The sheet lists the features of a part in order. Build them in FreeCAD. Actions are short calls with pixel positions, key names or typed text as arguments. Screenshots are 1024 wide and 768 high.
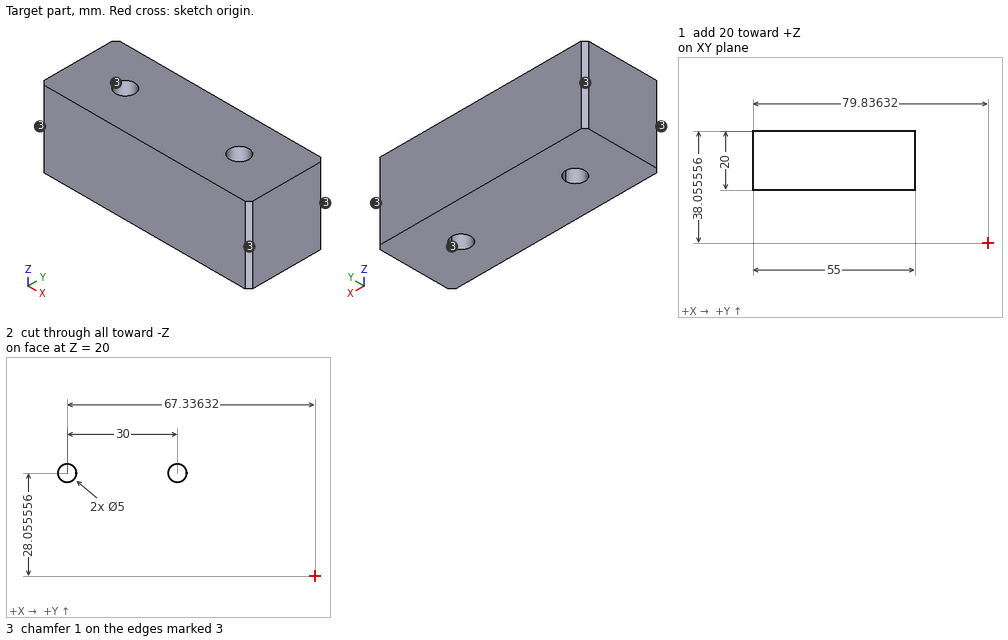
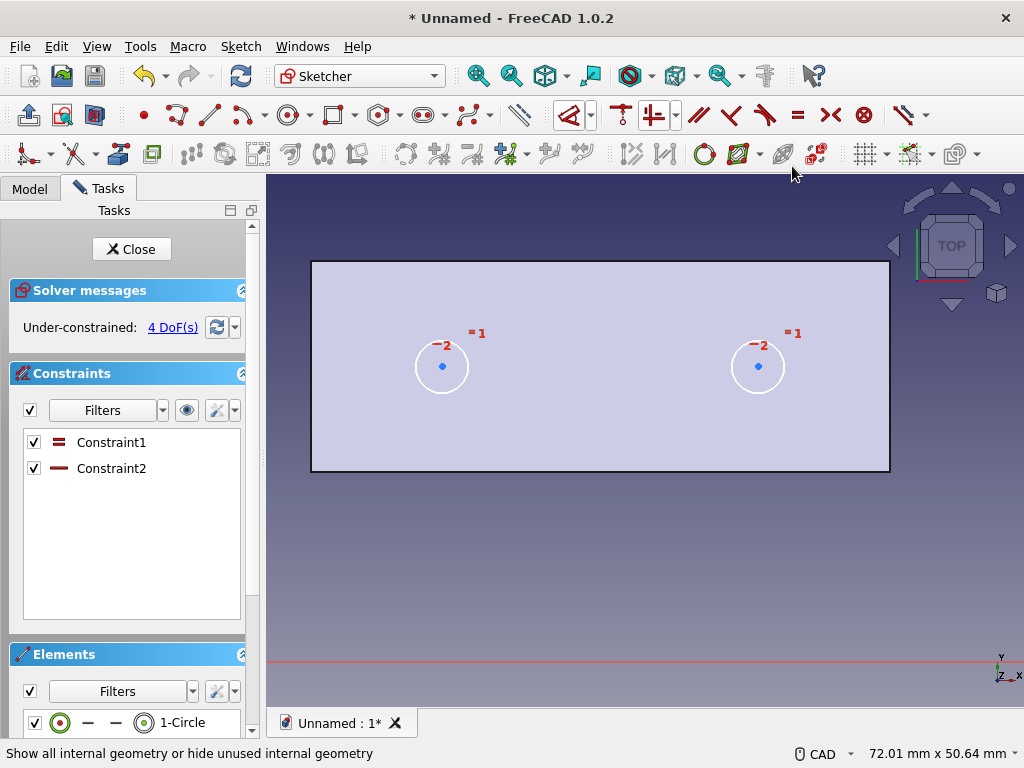
click(460, 348)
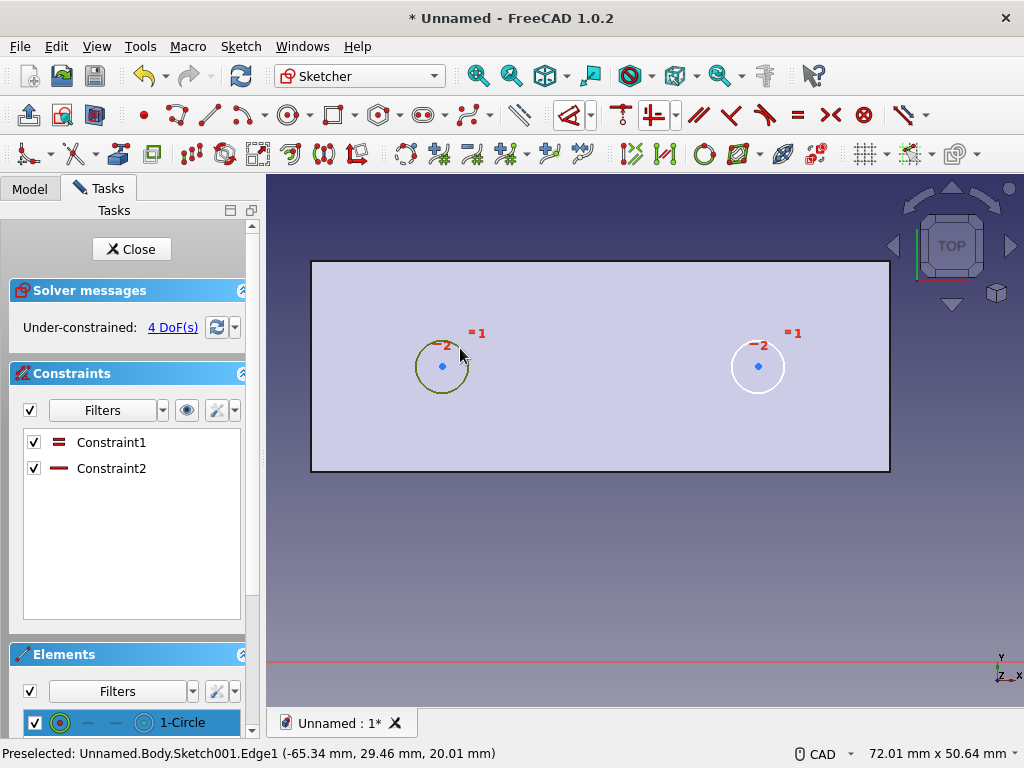
key(k)
key(o)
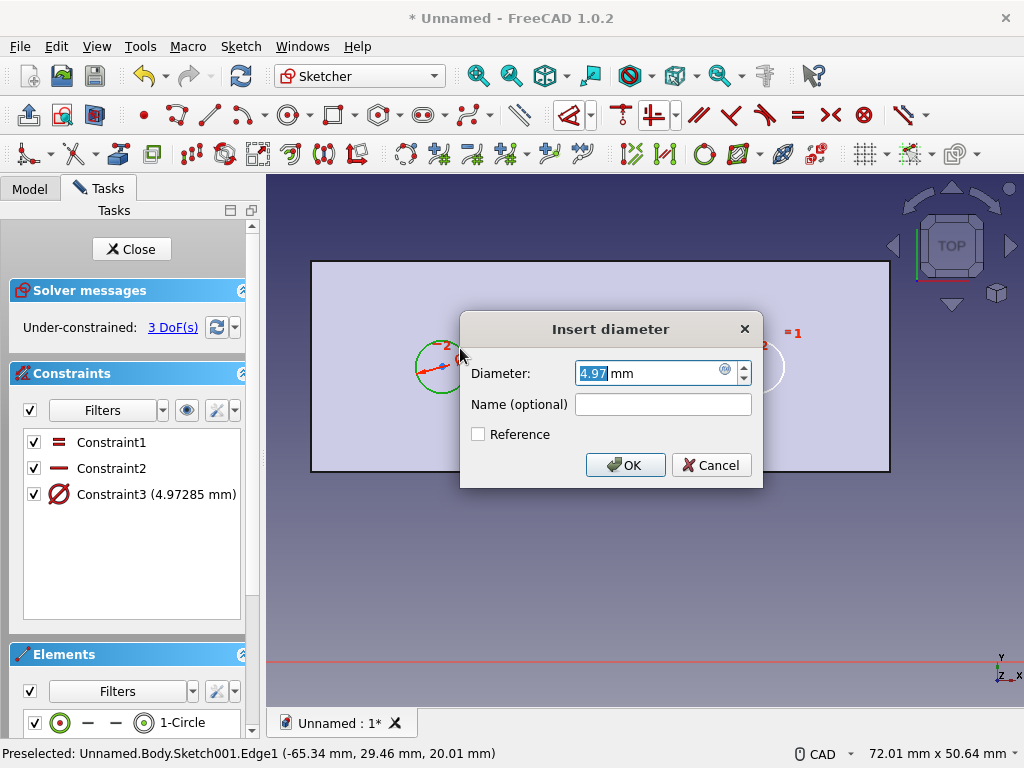
text(5)
key(Return)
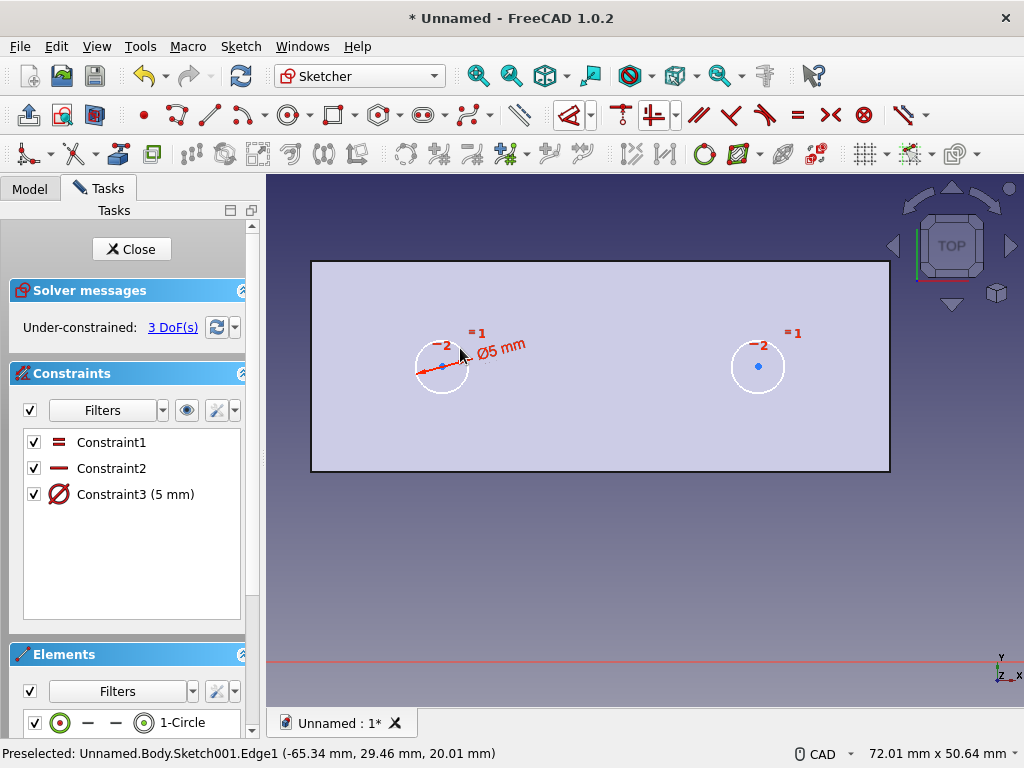
click(442, 367)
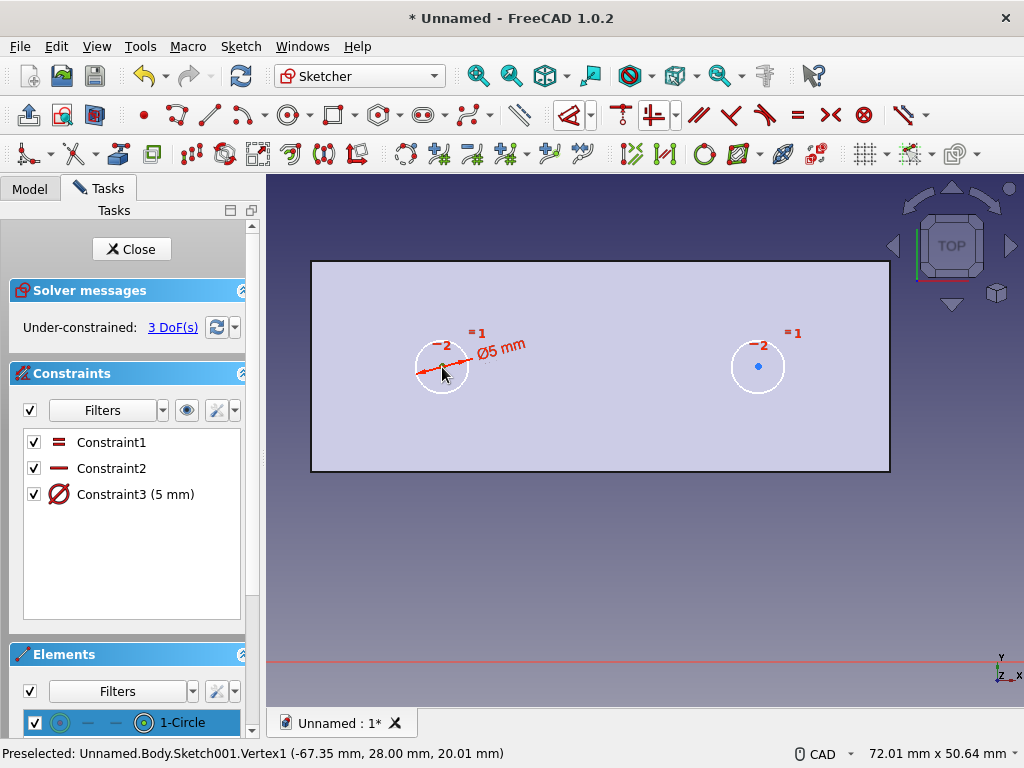
click(758, 367)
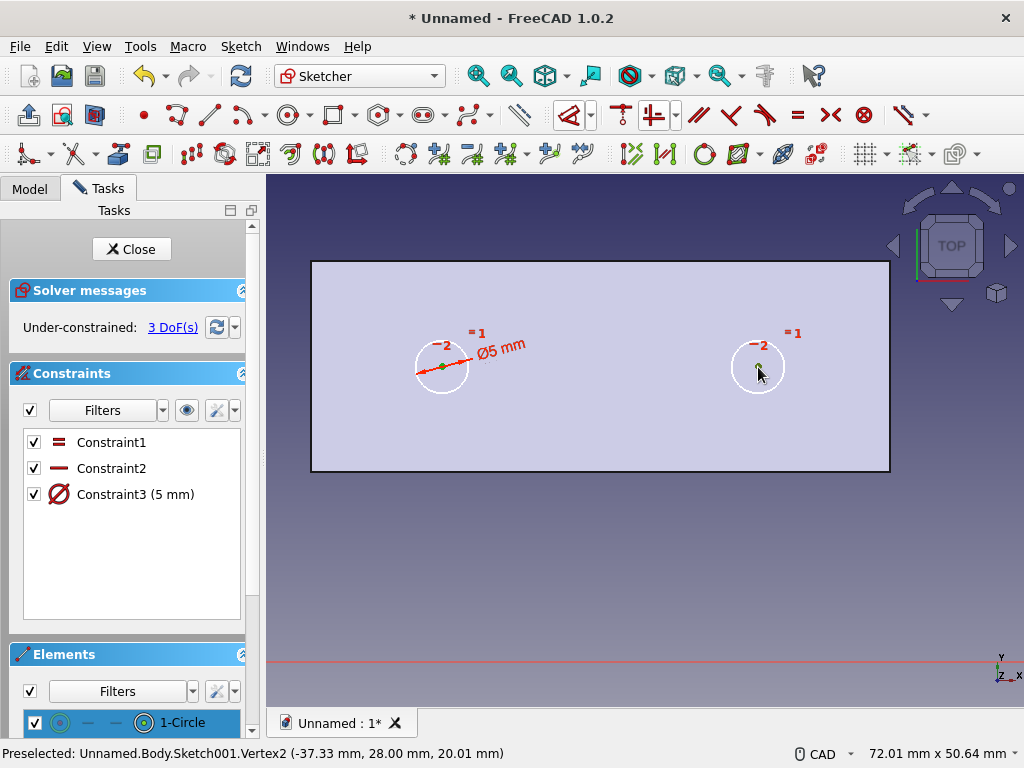
click(590, 116)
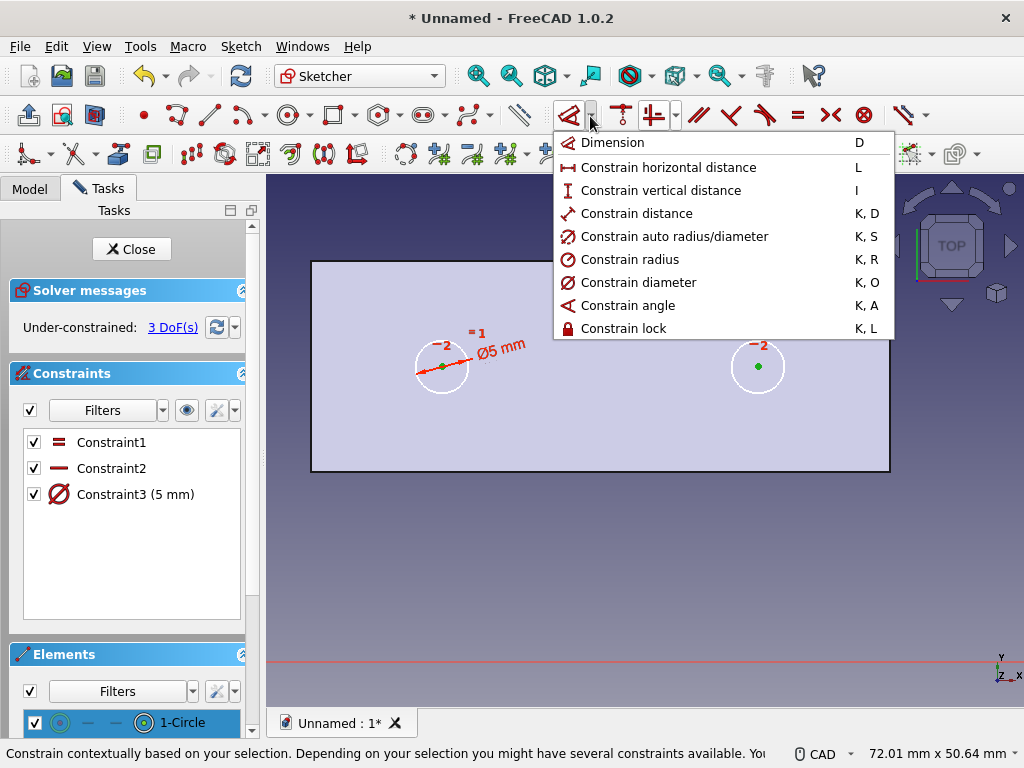
click(724, 168)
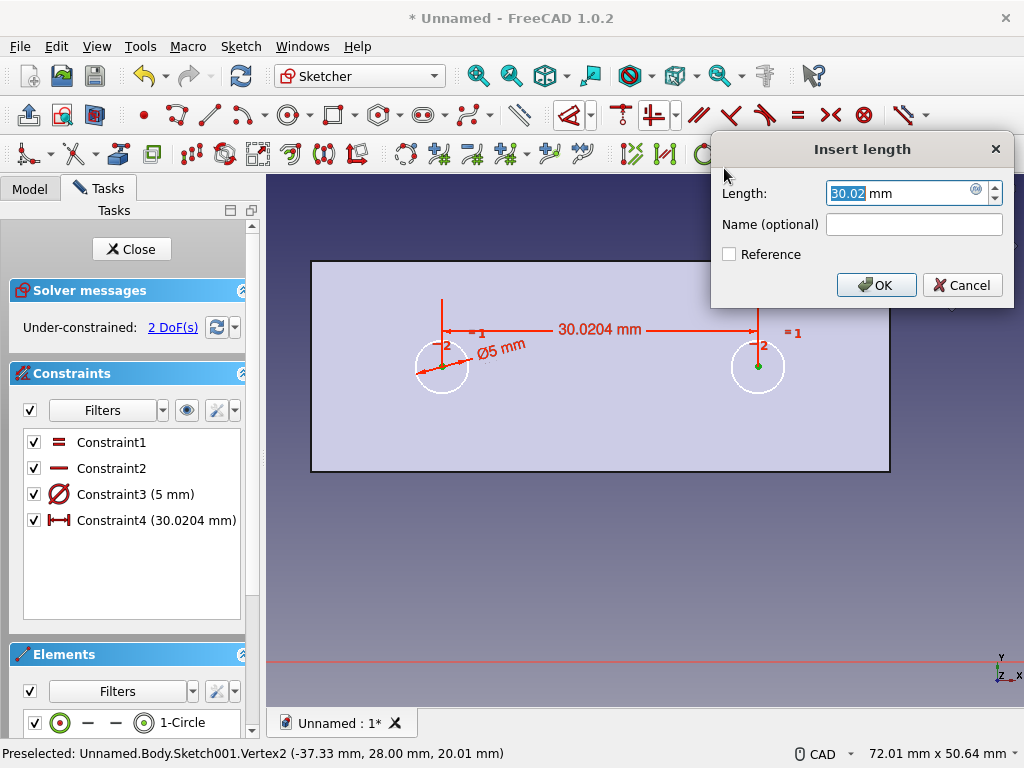
text(30)
key(Return)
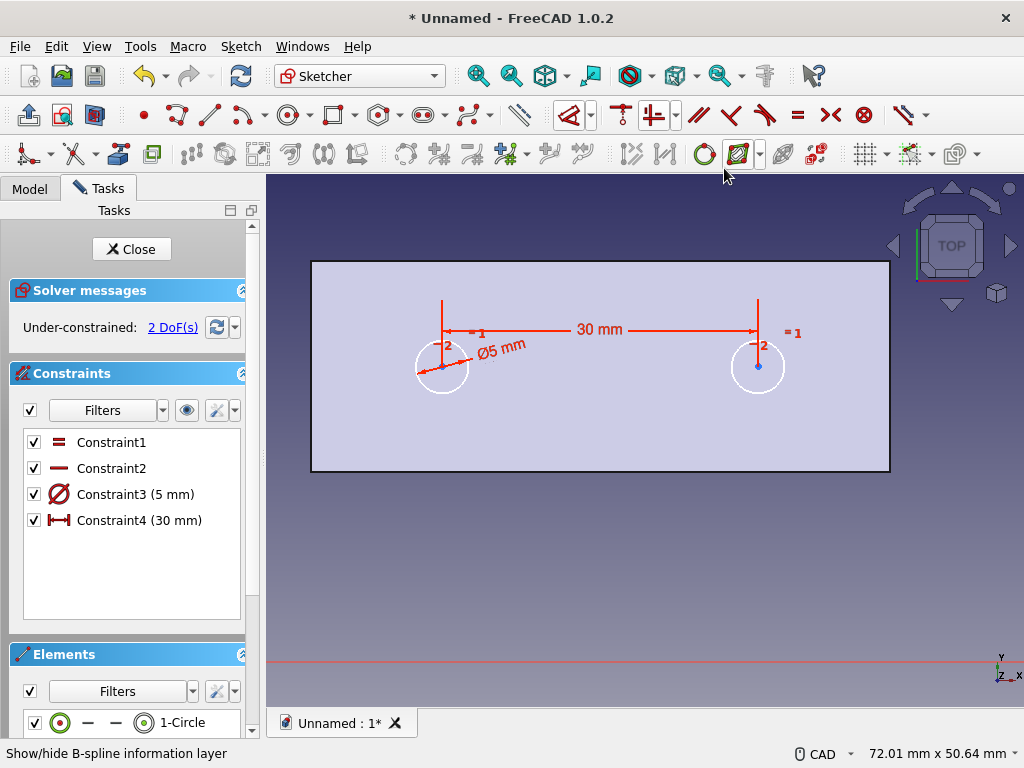
click(442, 367)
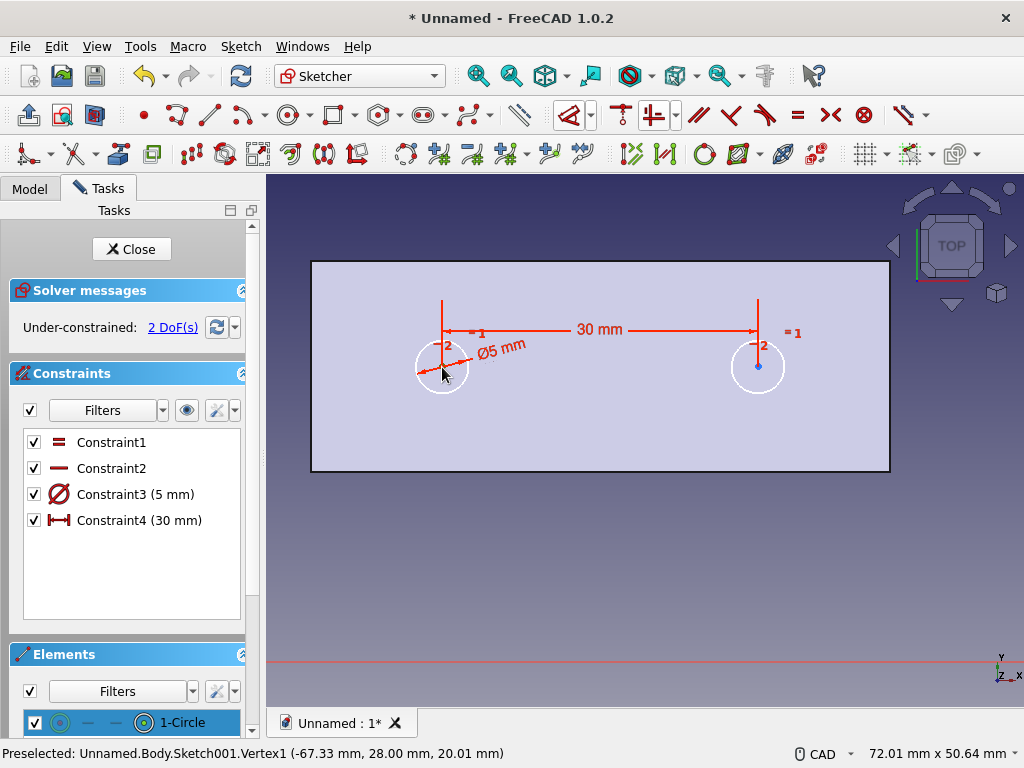
click(590, 116)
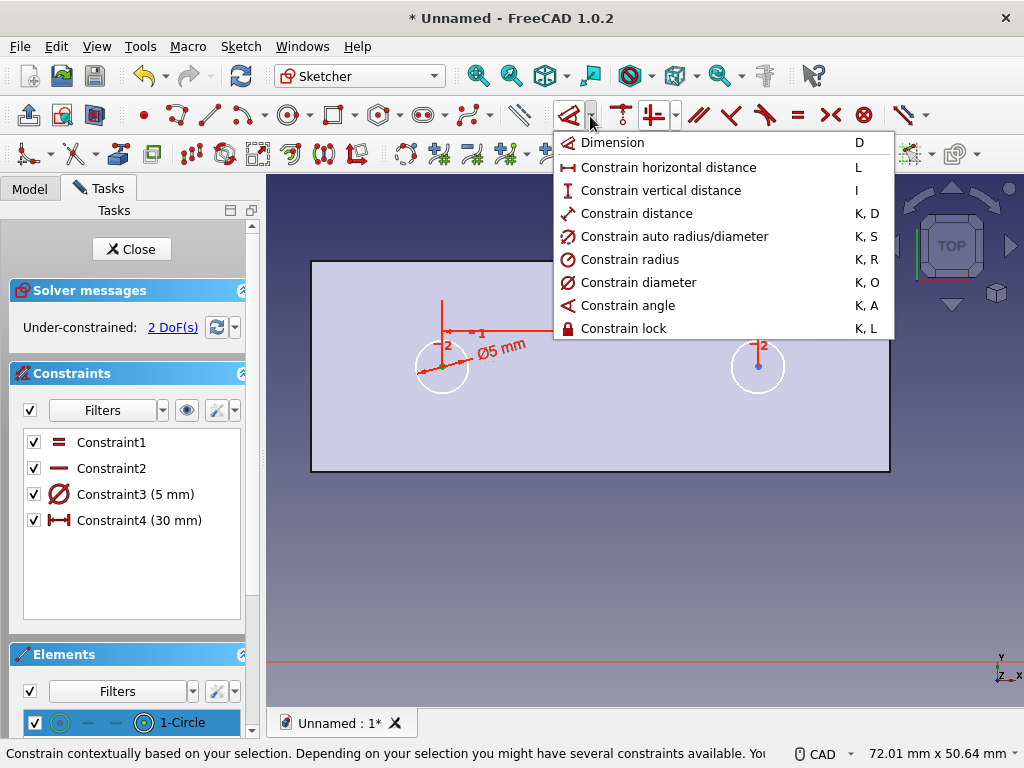
click(724, 168)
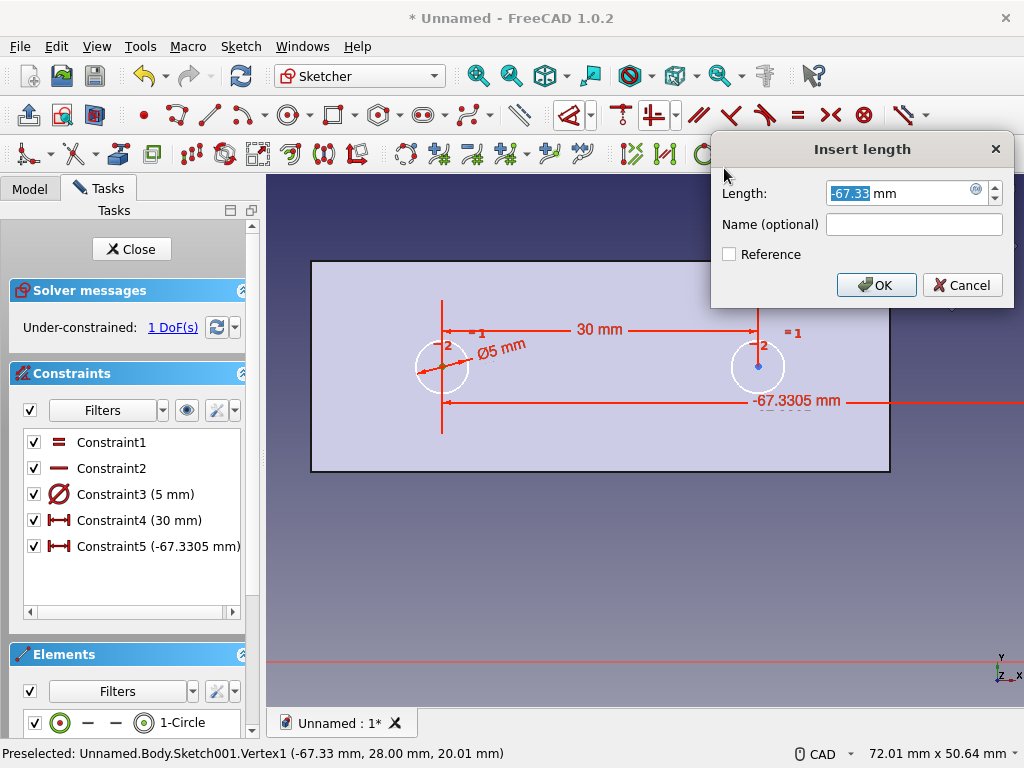
text(-67.33632)
key(Return)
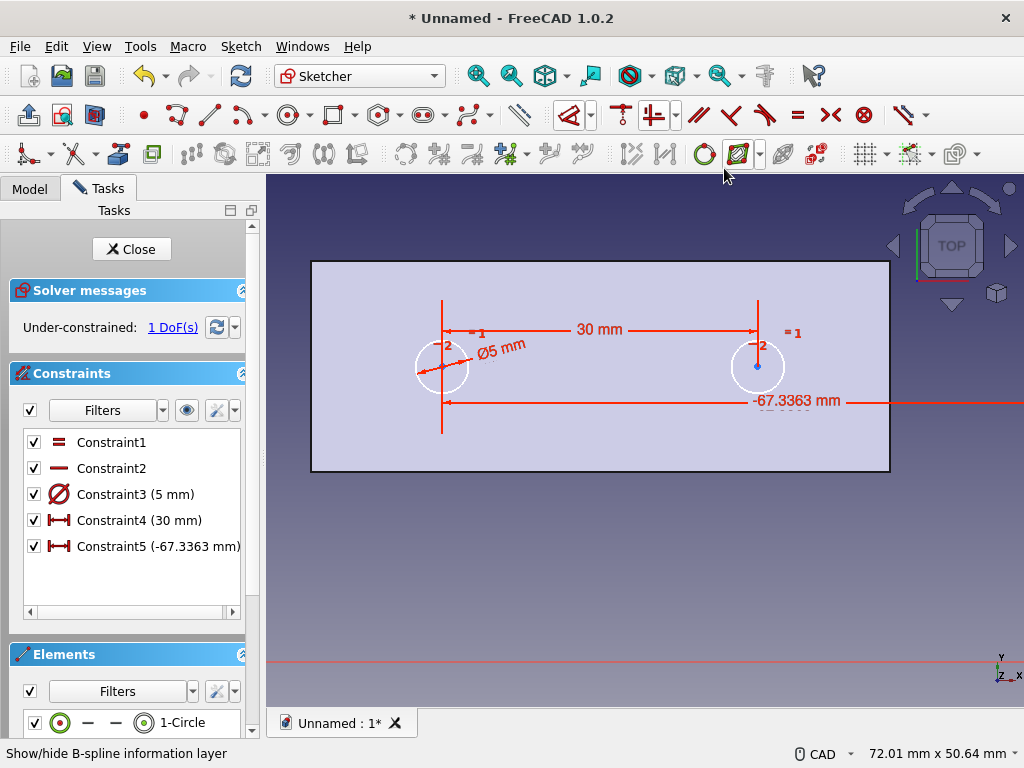
click(442, 367)